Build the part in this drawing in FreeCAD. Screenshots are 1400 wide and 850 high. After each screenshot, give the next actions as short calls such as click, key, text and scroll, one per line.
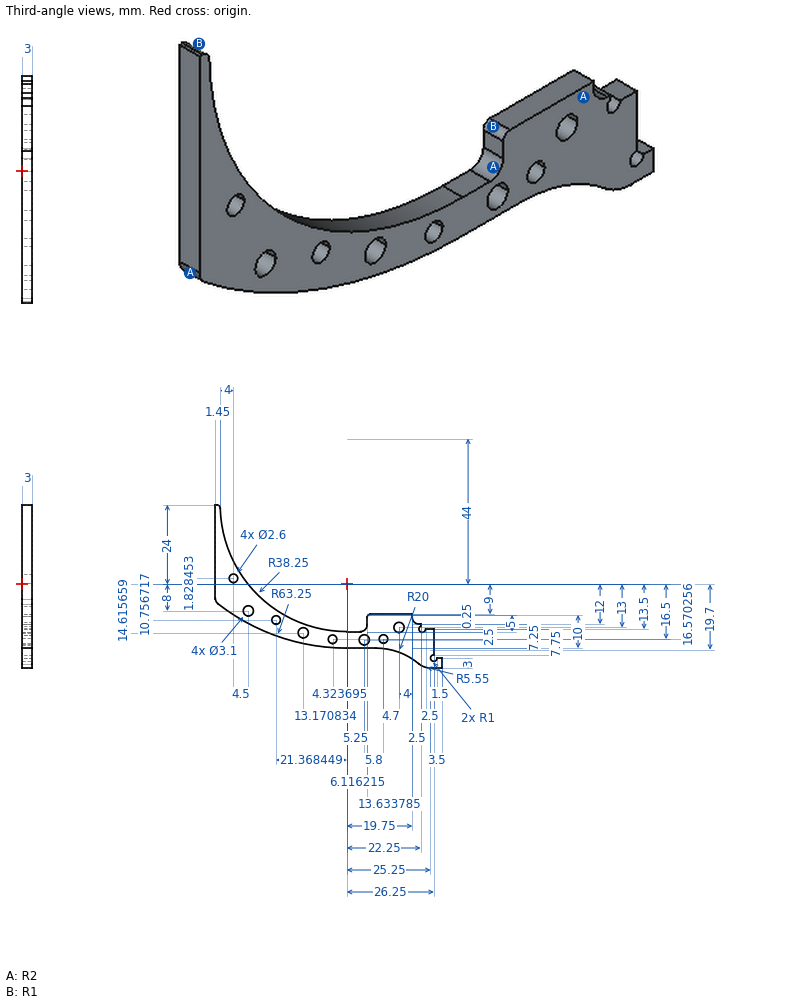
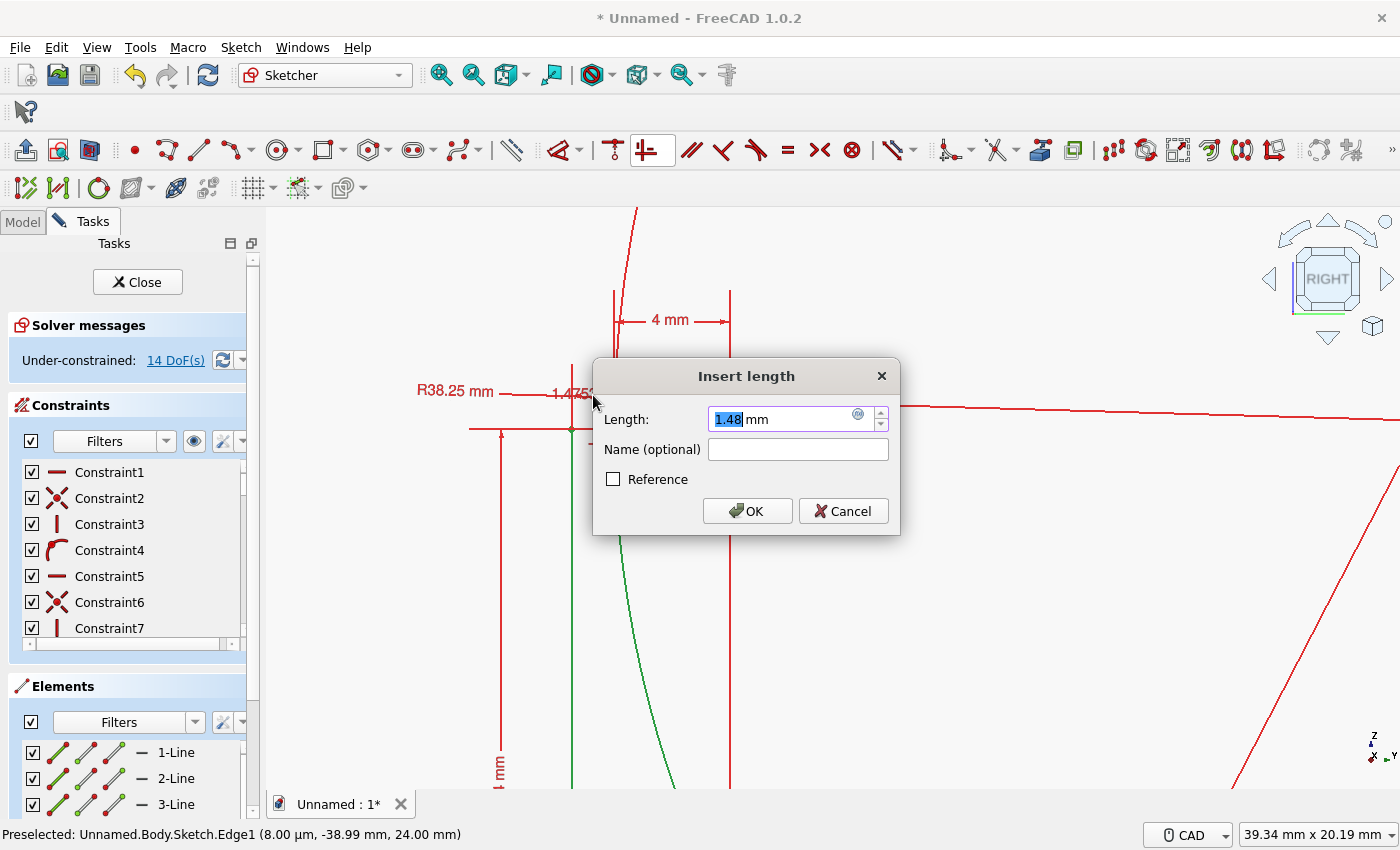
text(1.45)
key(Return)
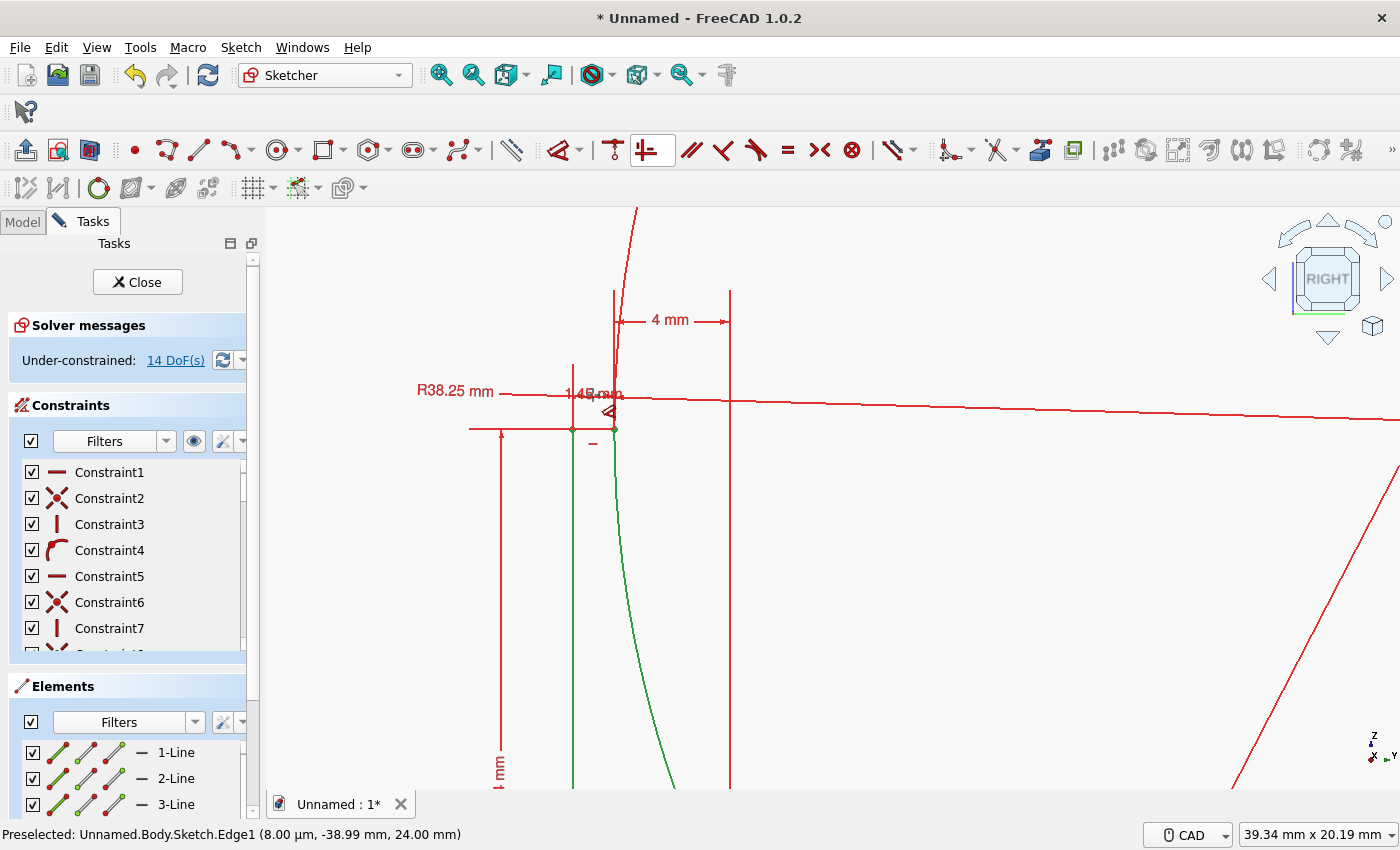
scroll(478, 259, down, 6)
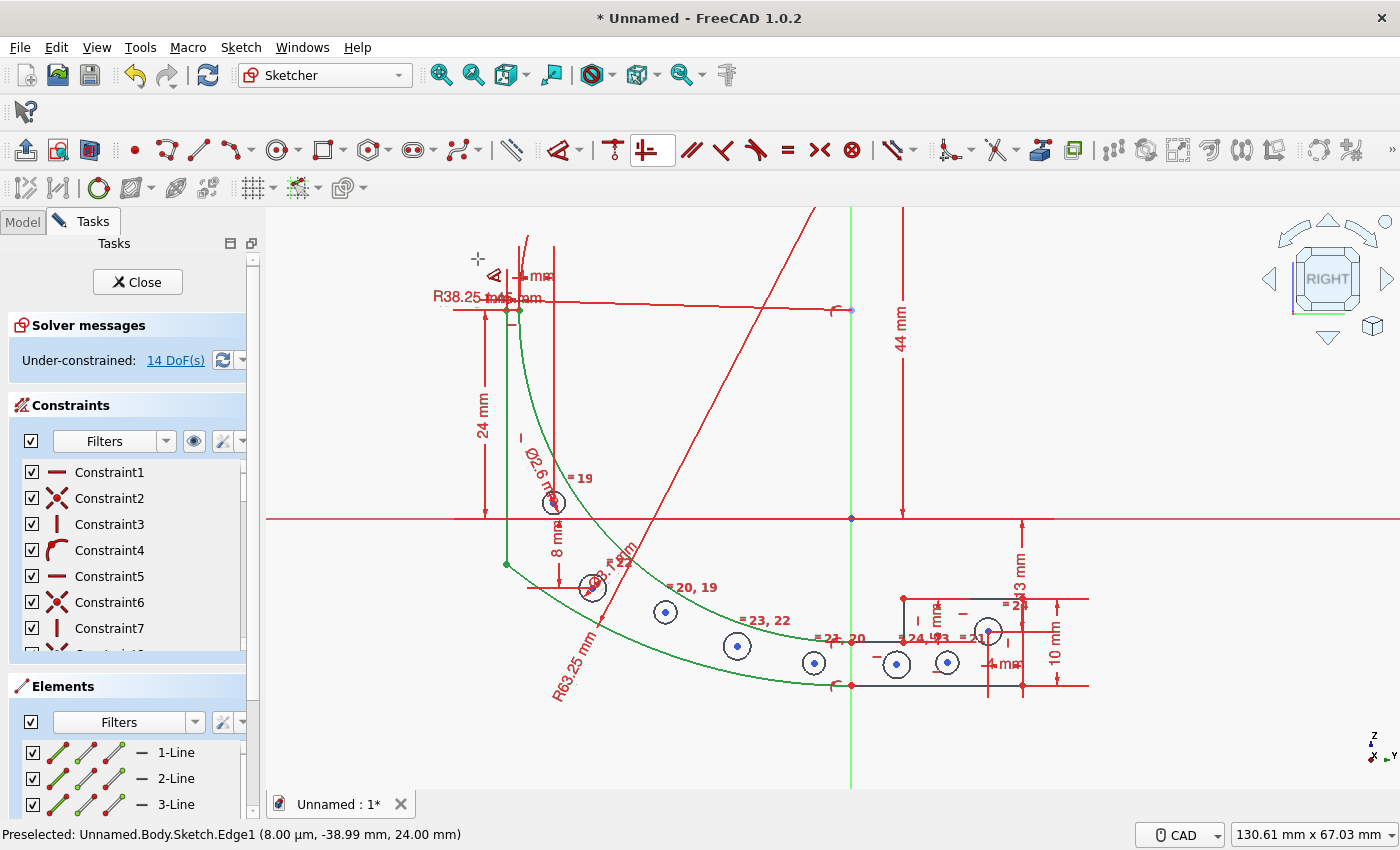
click(897, 665)
click(874, 699)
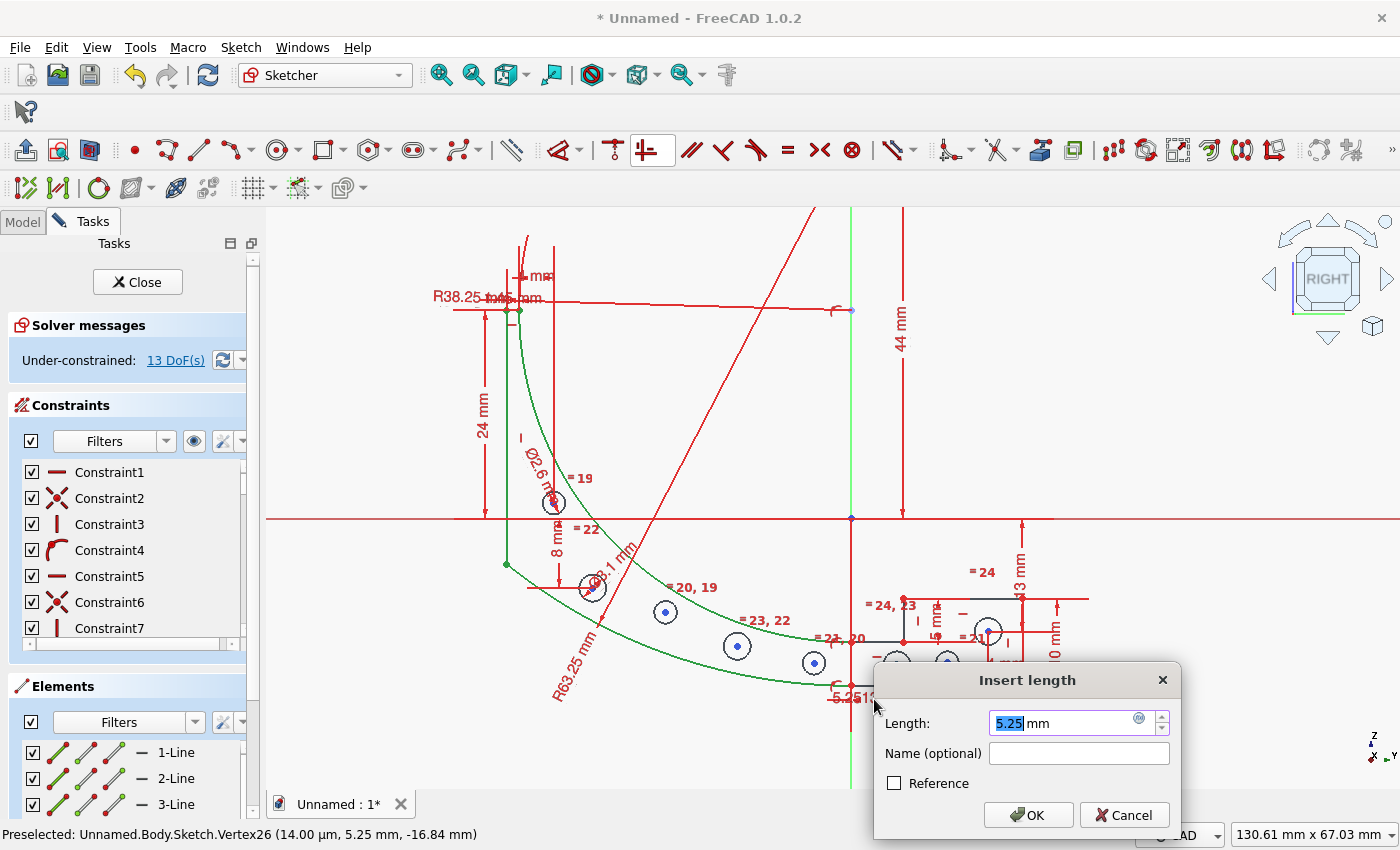
text(5.25)
key(Return)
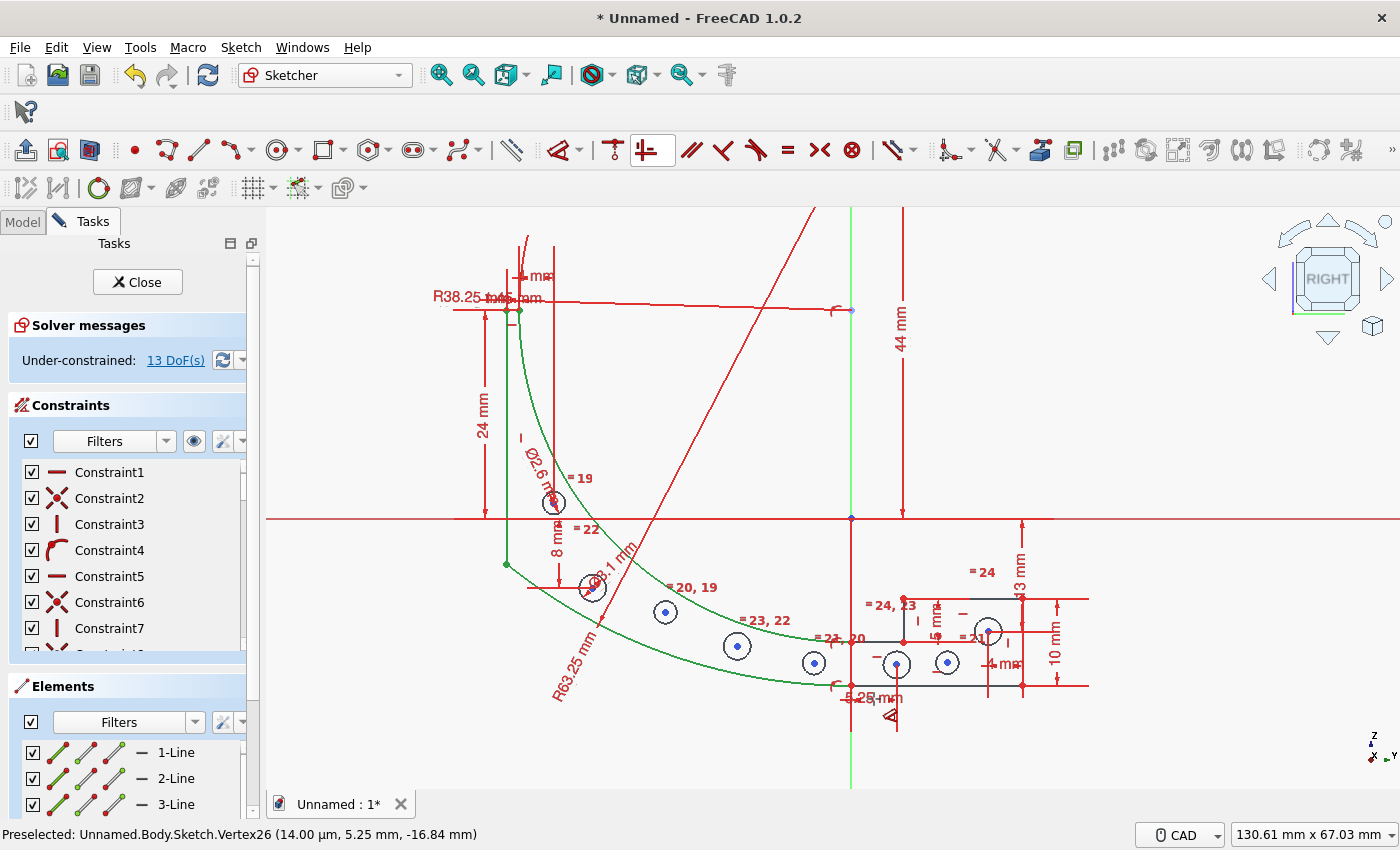
click(947, 663)
click(981, 540)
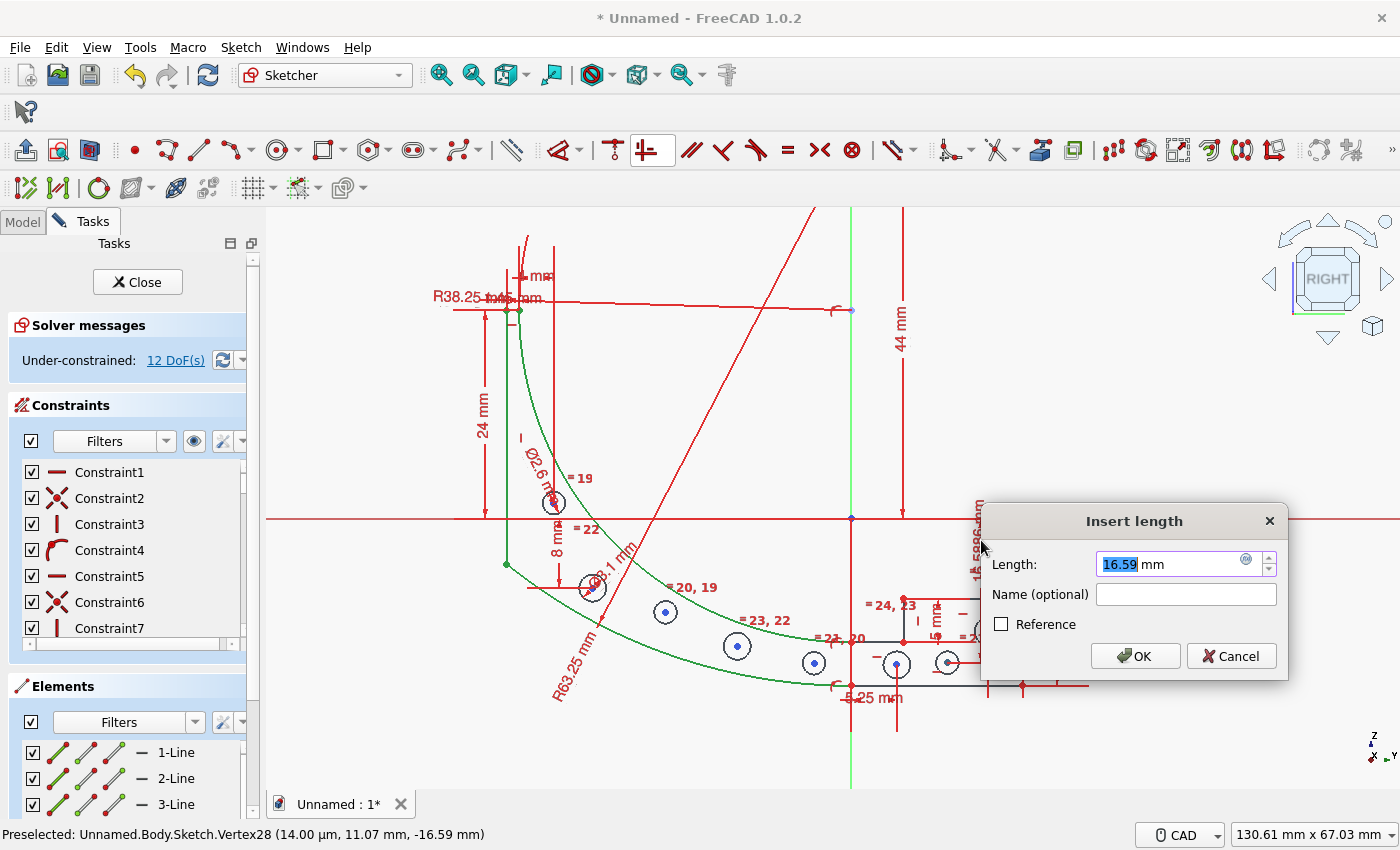
text(16.5)
key(Return)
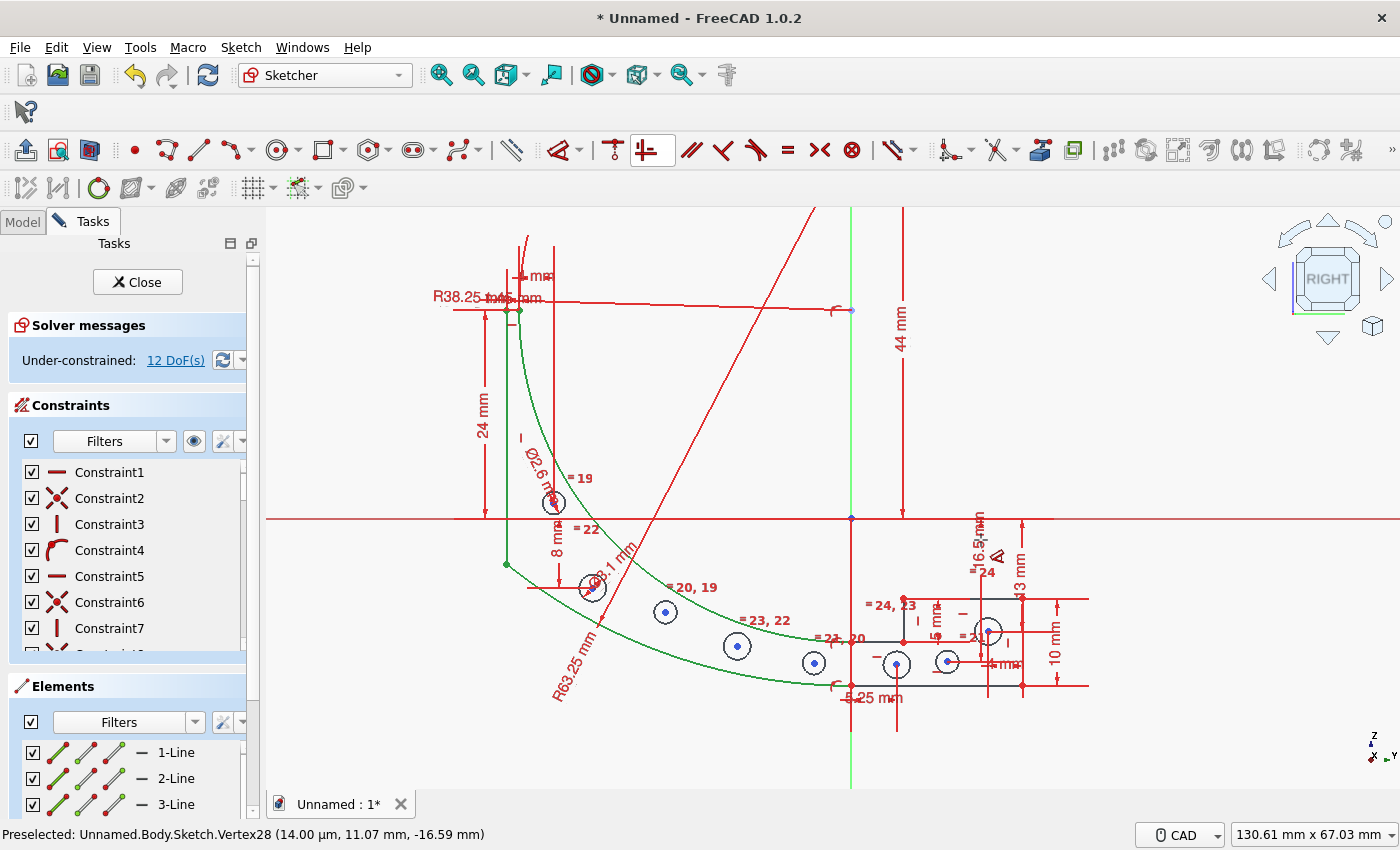
click(554, 503)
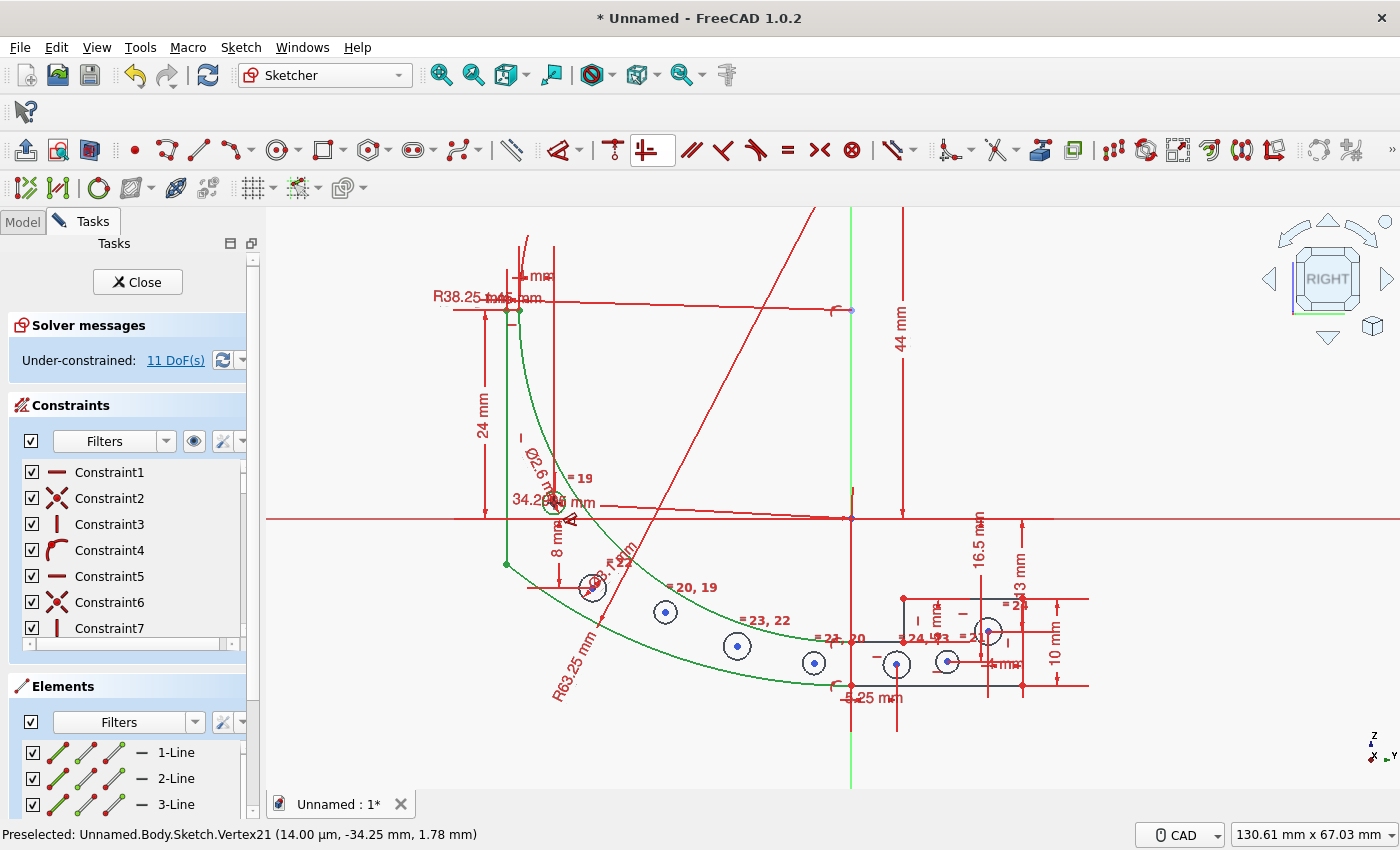
click(593, 588)
click(564, 622)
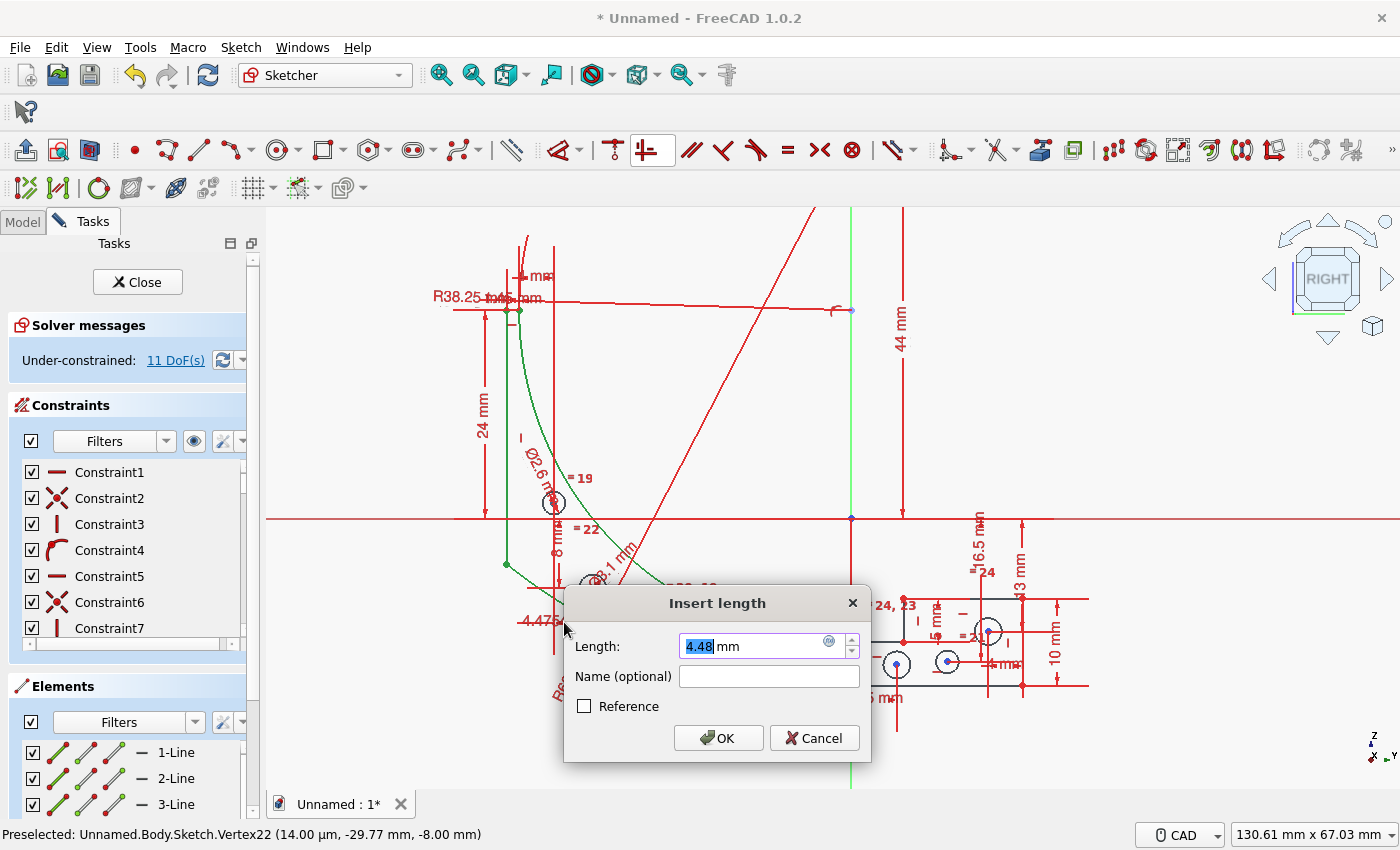
text(4.5)
key(Return)